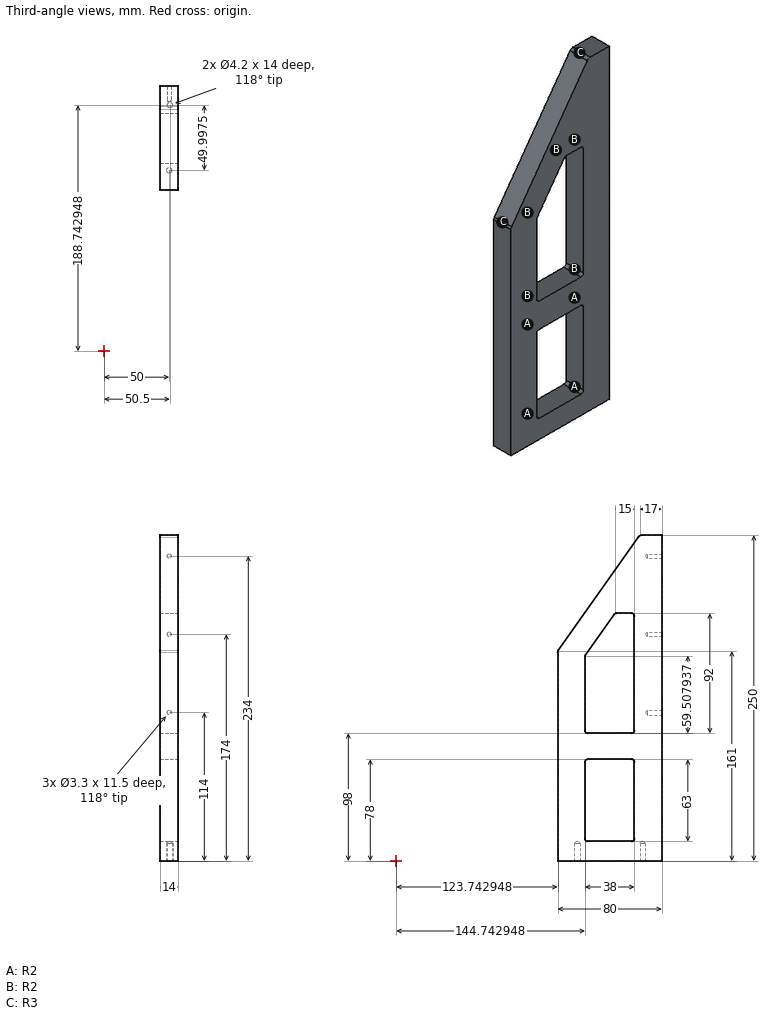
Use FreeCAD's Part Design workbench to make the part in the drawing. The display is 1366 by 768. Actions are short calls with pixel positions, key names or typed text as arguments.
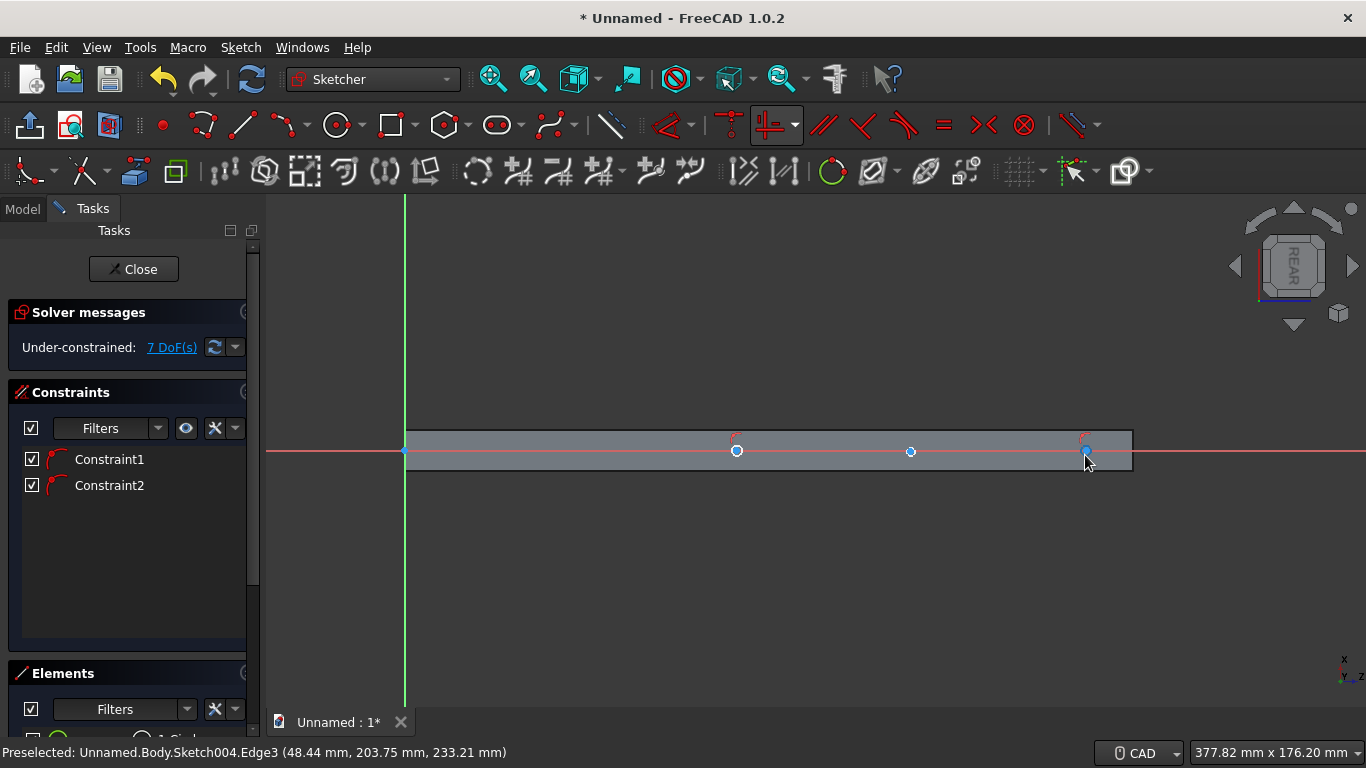
scroll(741, 447, up, 7)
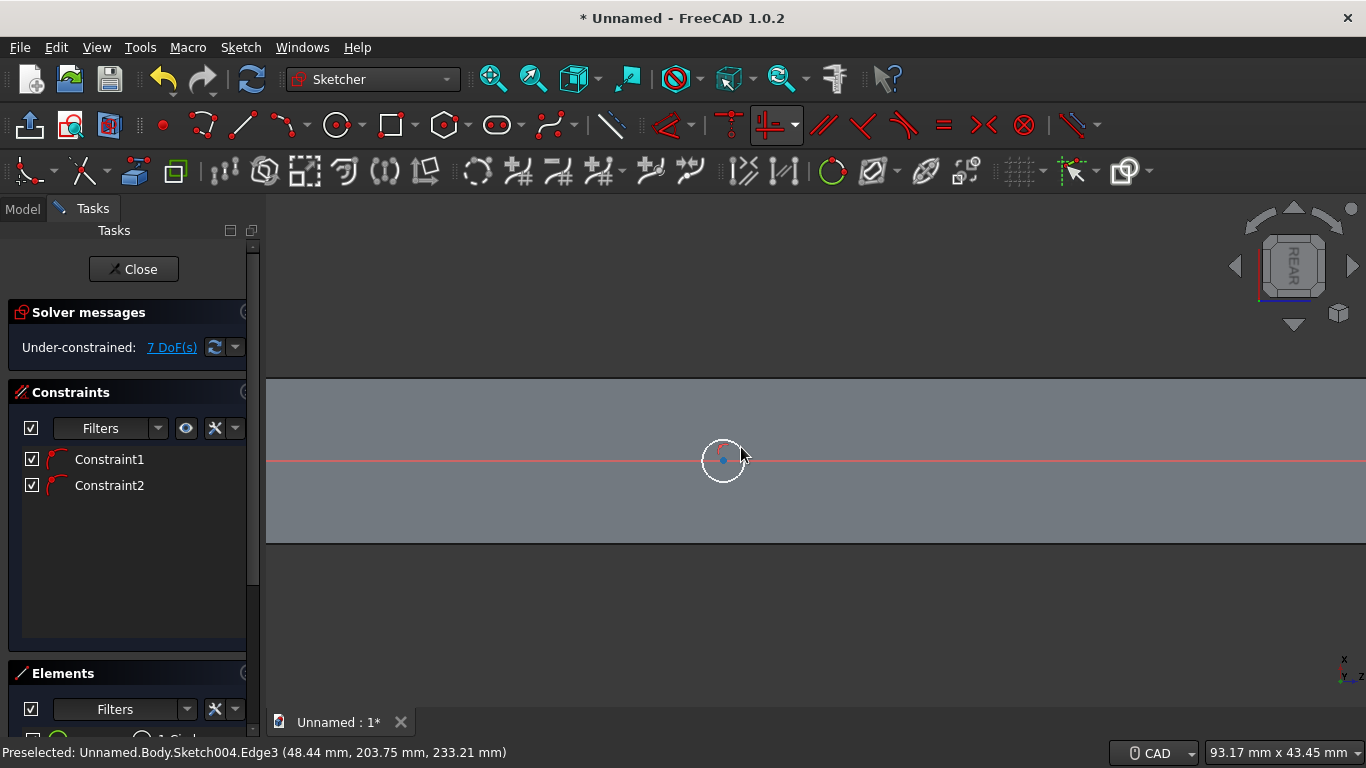
click(738, 446)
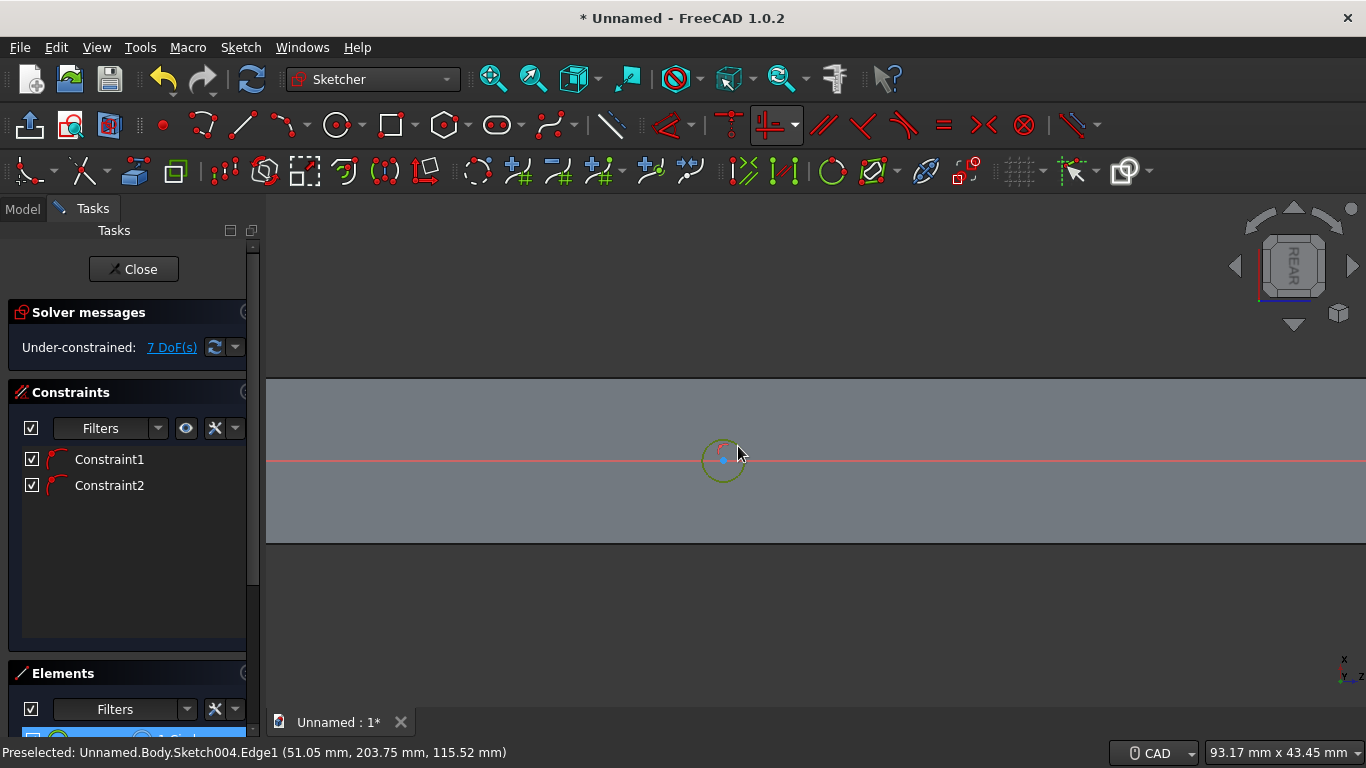
scroll(741, 447, down, 7)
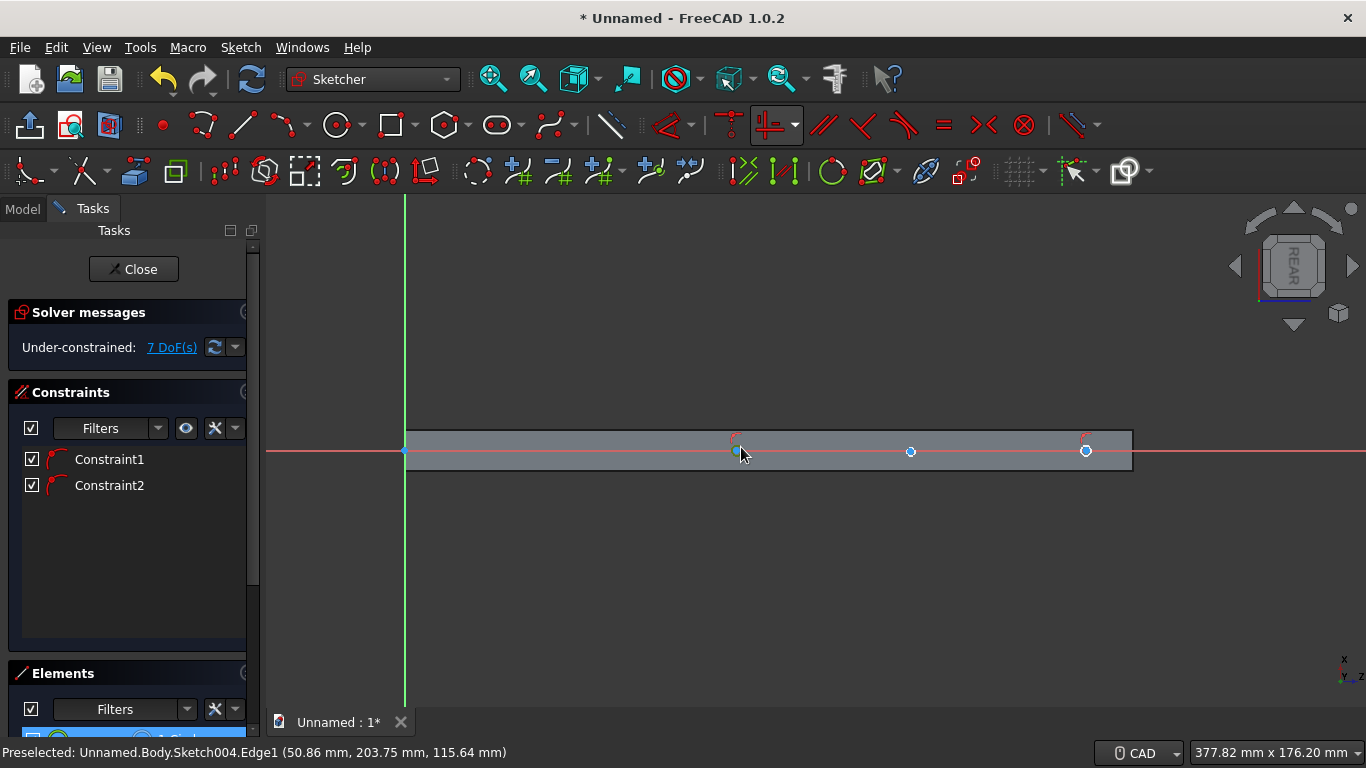
scroll(908, 455, up, 7)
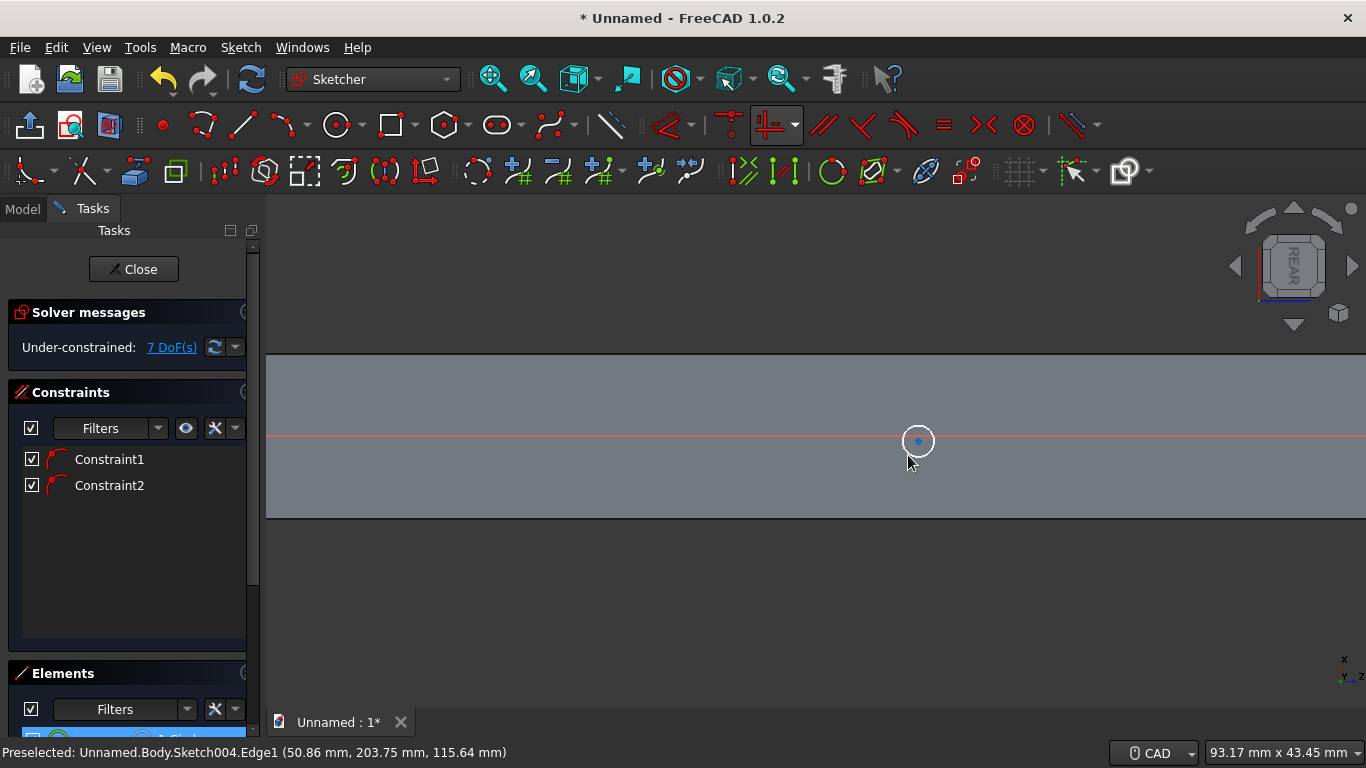
click(907, 452)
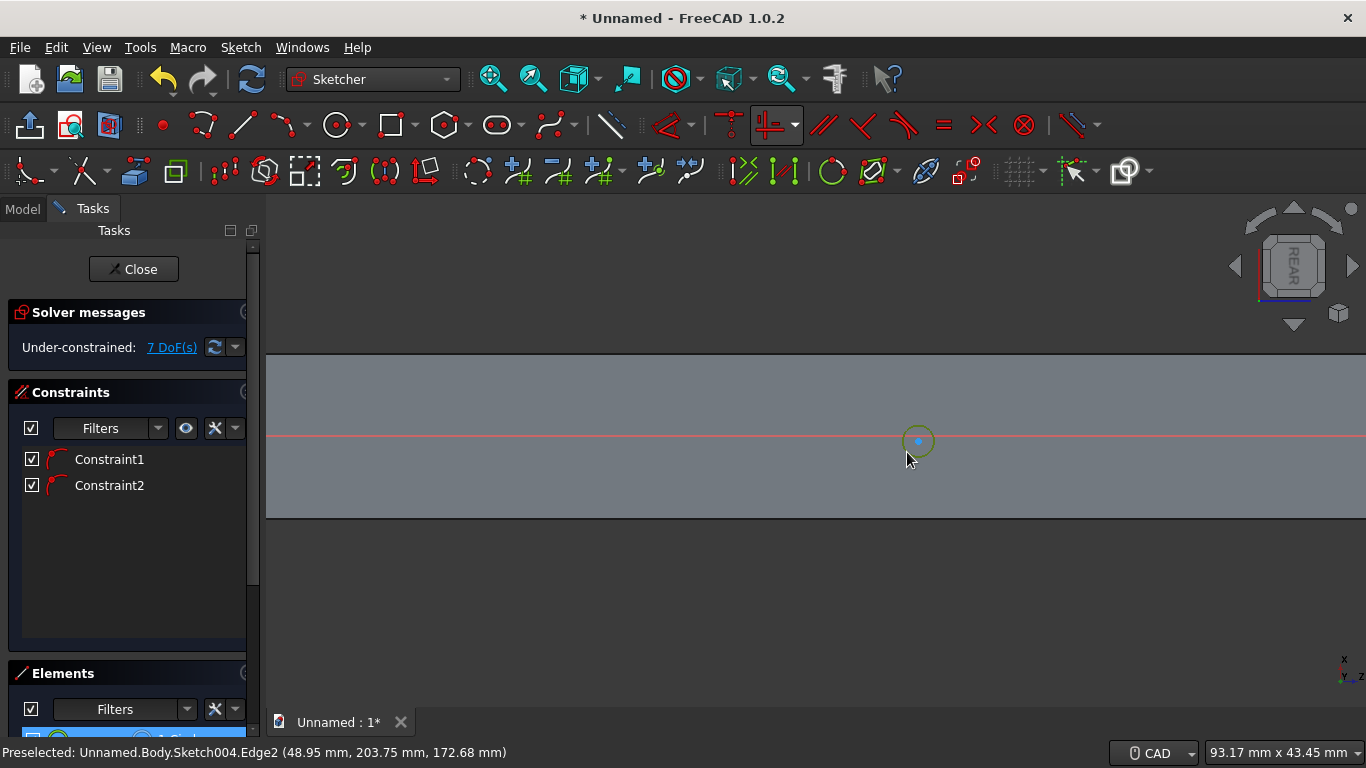
scroll(908, 455, down, 7)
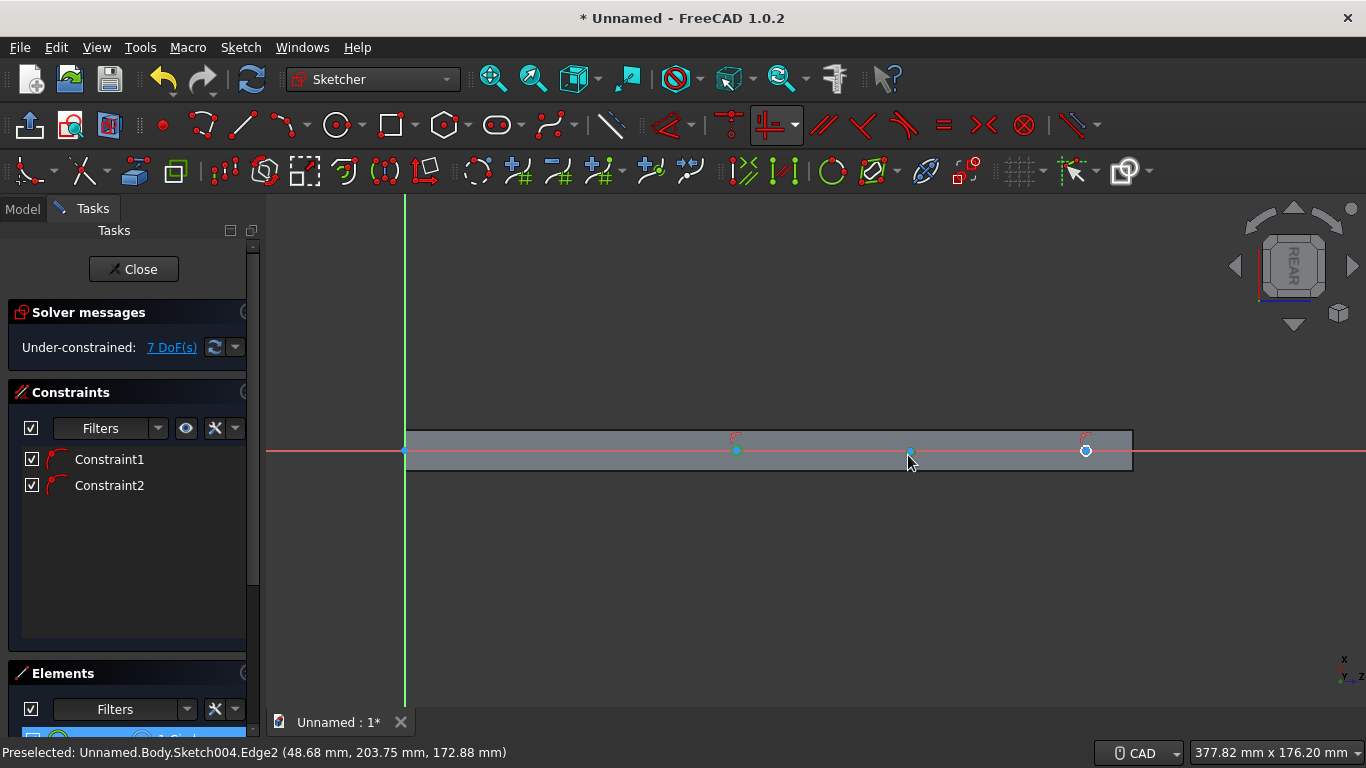
scroll(1090, 447, up, 7)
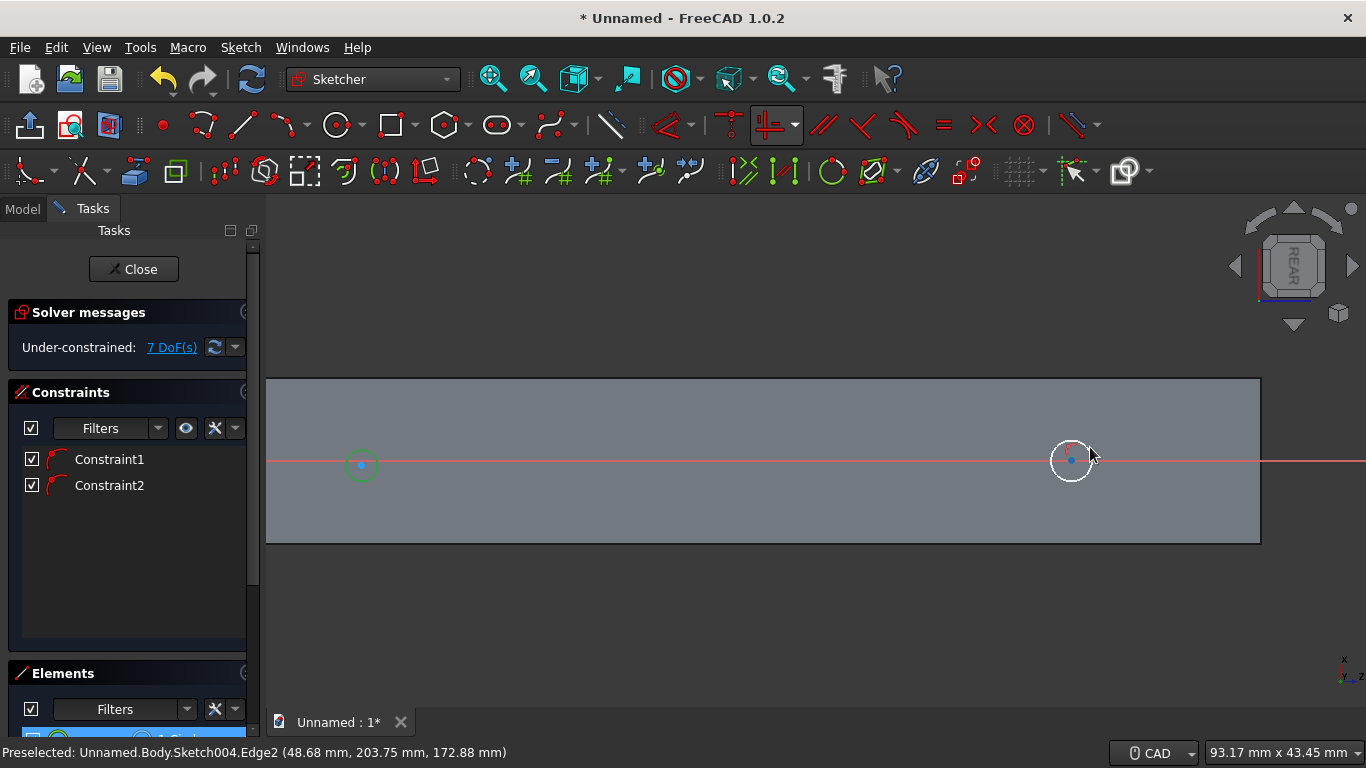
click(1086, 446)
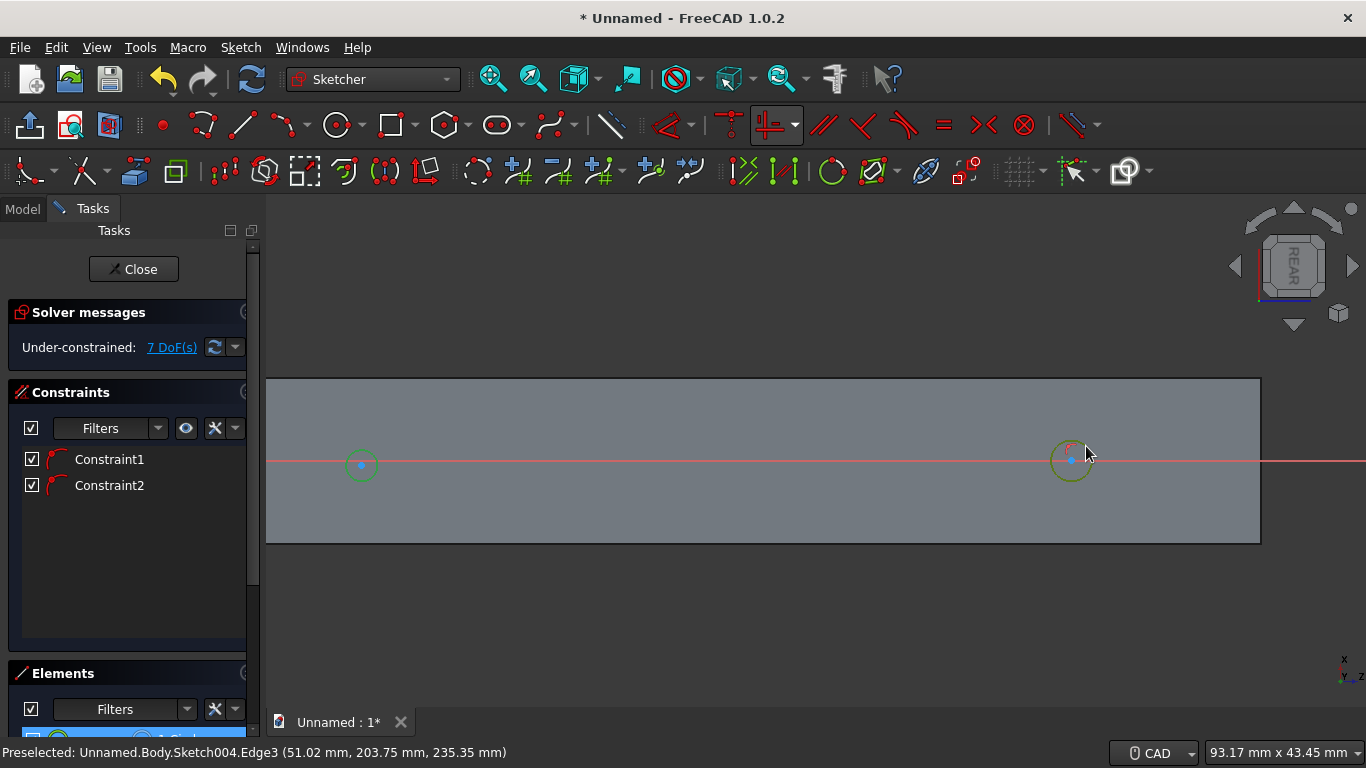
click(944, 126)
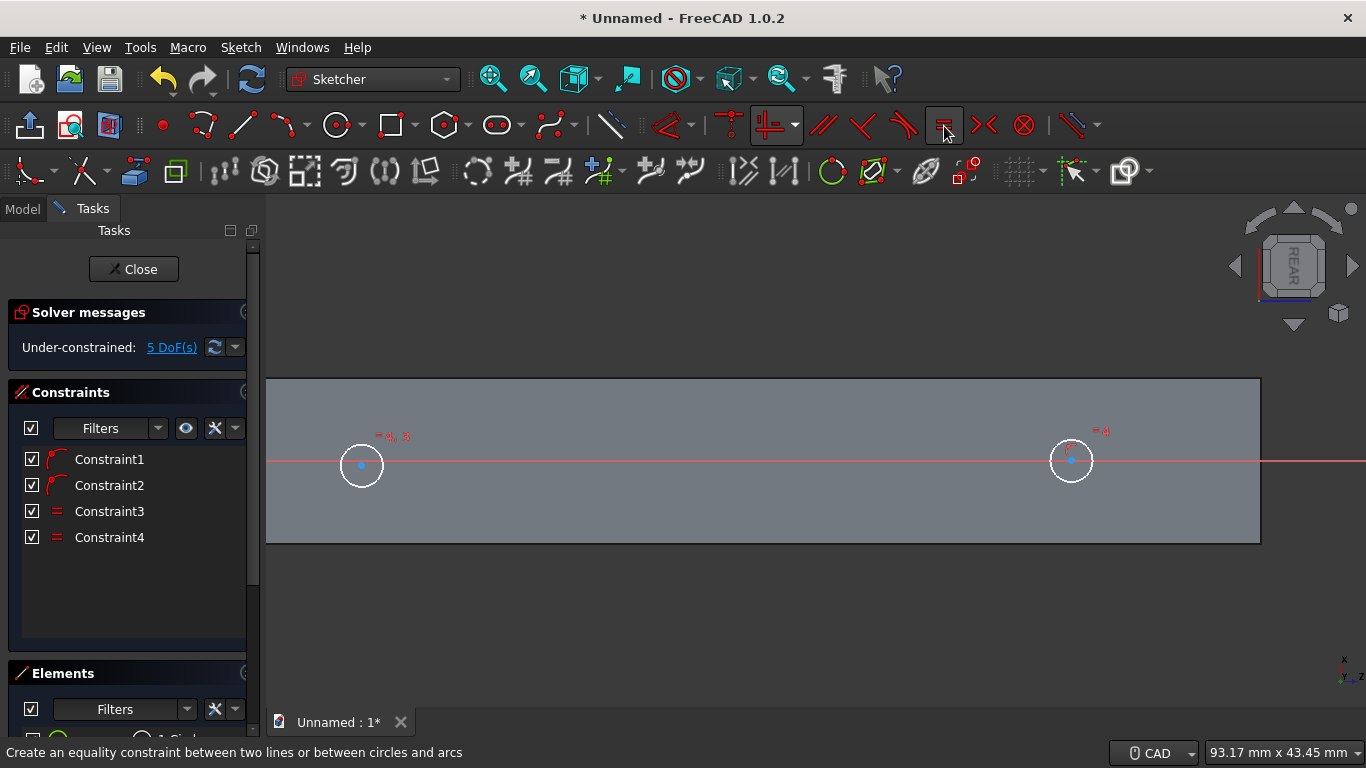
scroll(1090, 447, down, 7)